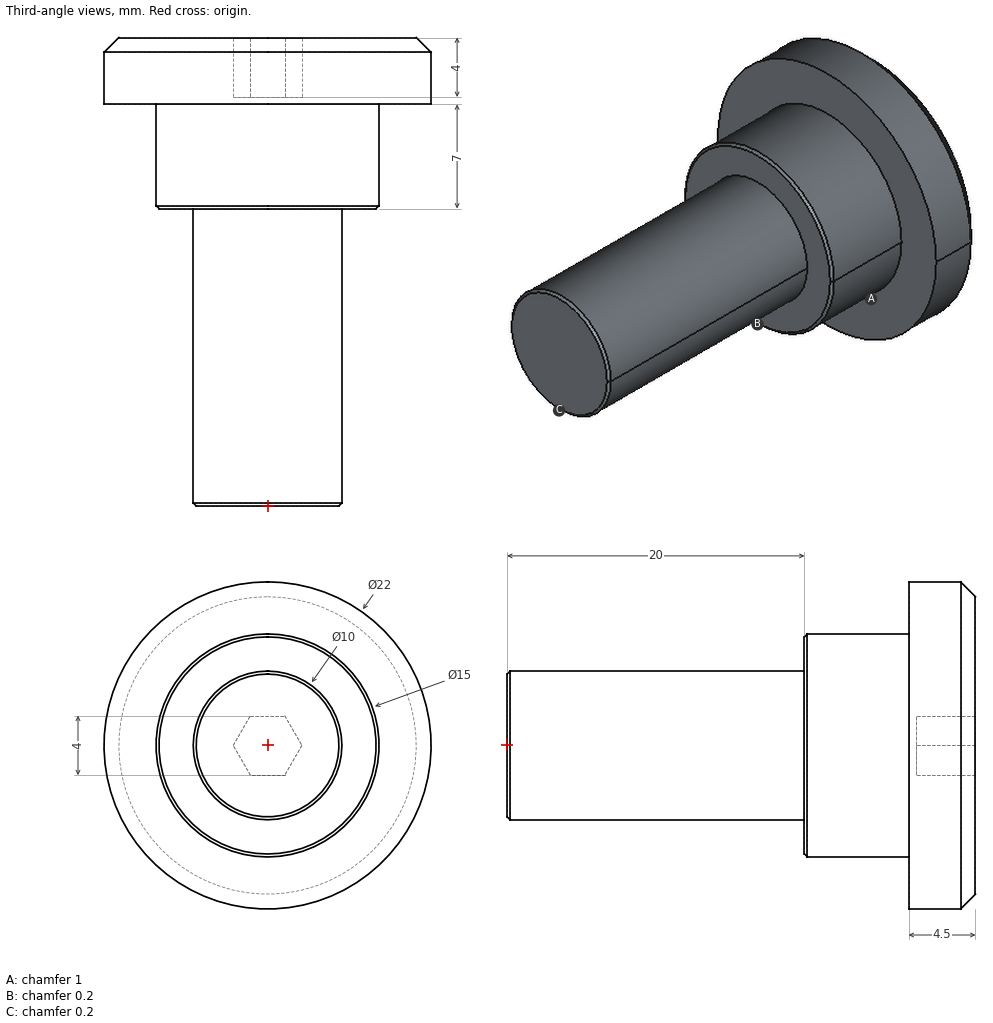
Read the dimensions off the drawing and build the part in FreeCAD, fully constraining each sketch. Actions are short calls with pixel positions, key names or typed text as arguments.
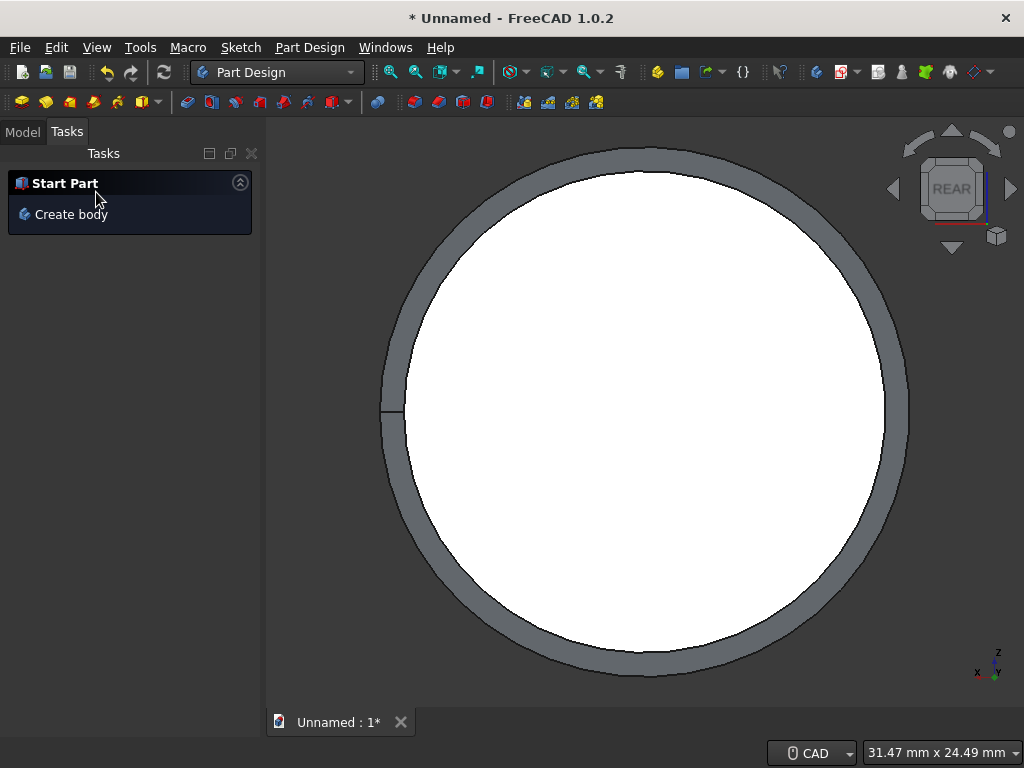
key(0)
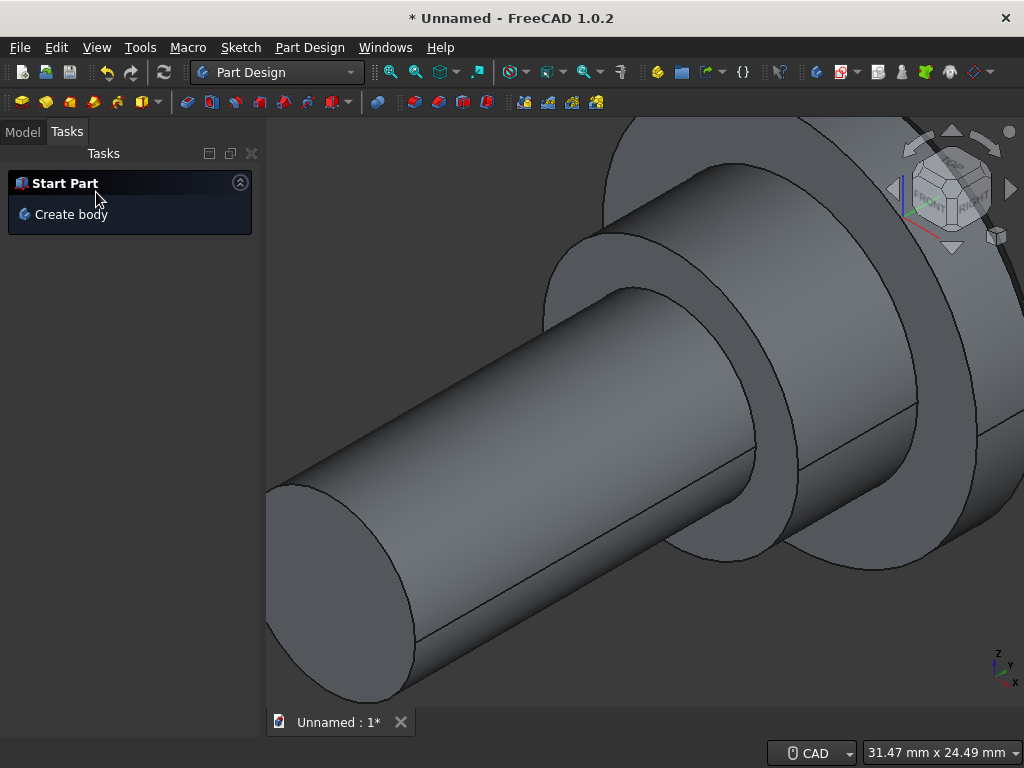
key(v)
key(f)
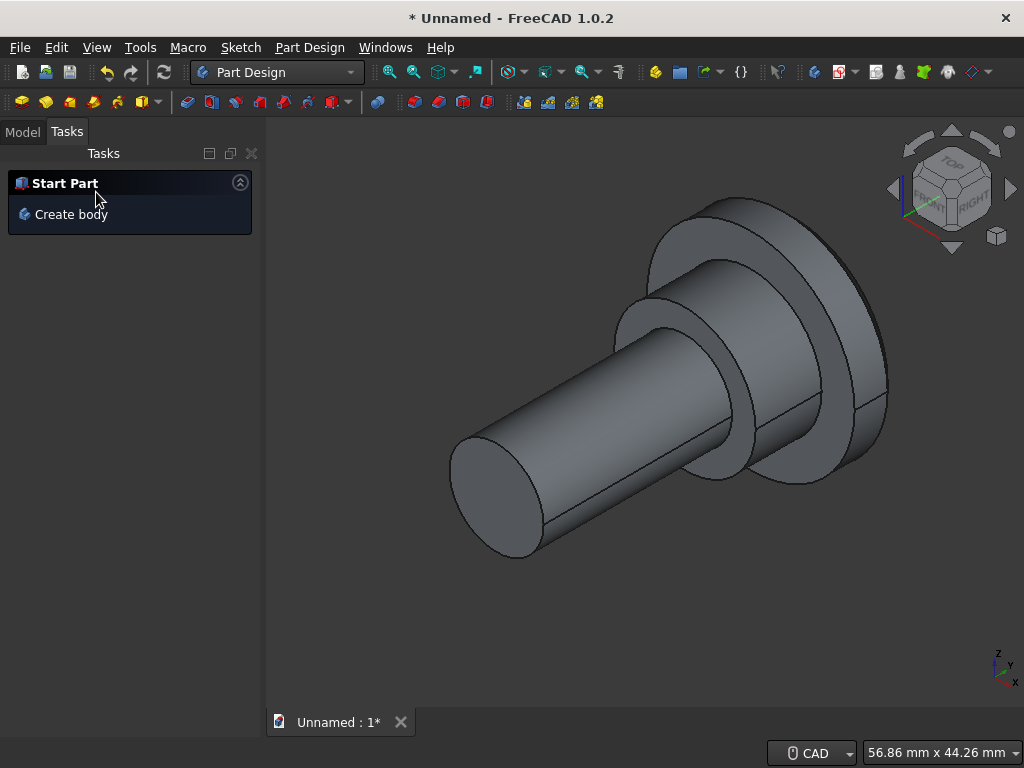
click(628, 307)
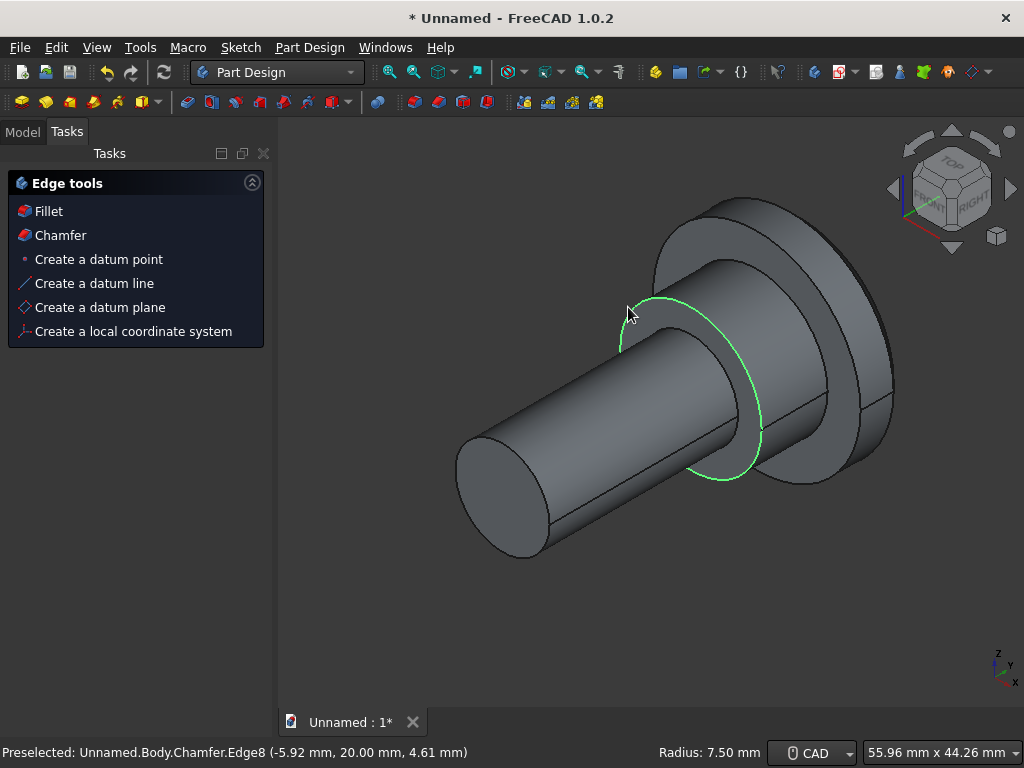
click(440, 102)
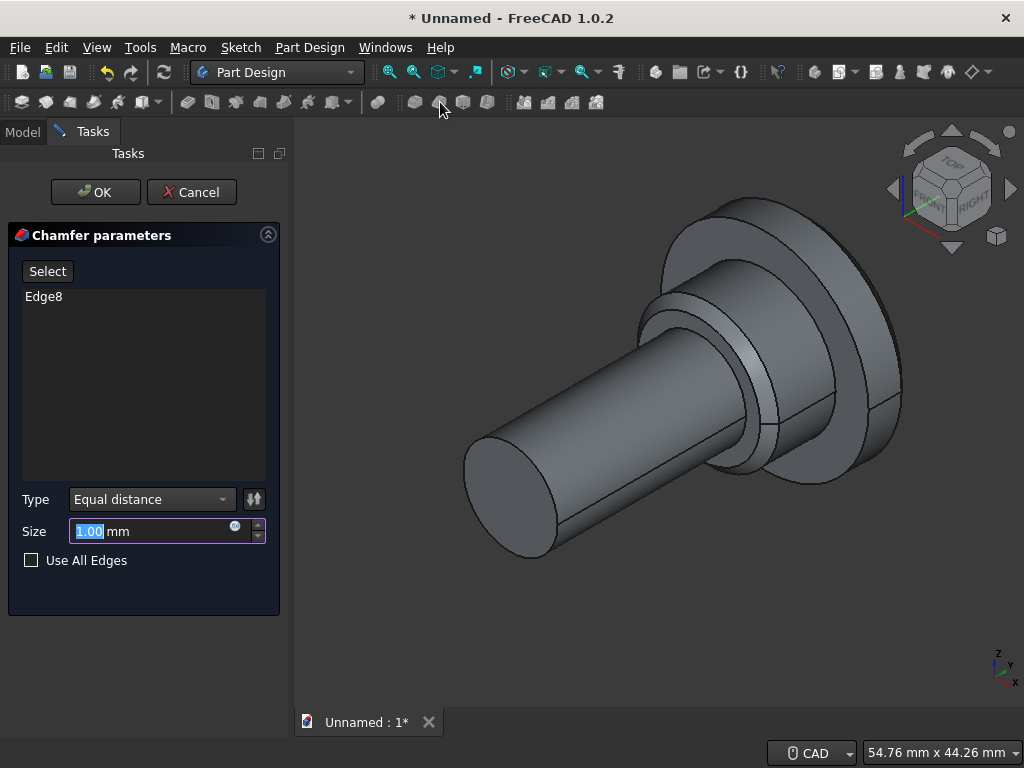
text(0.2)
key(Tab)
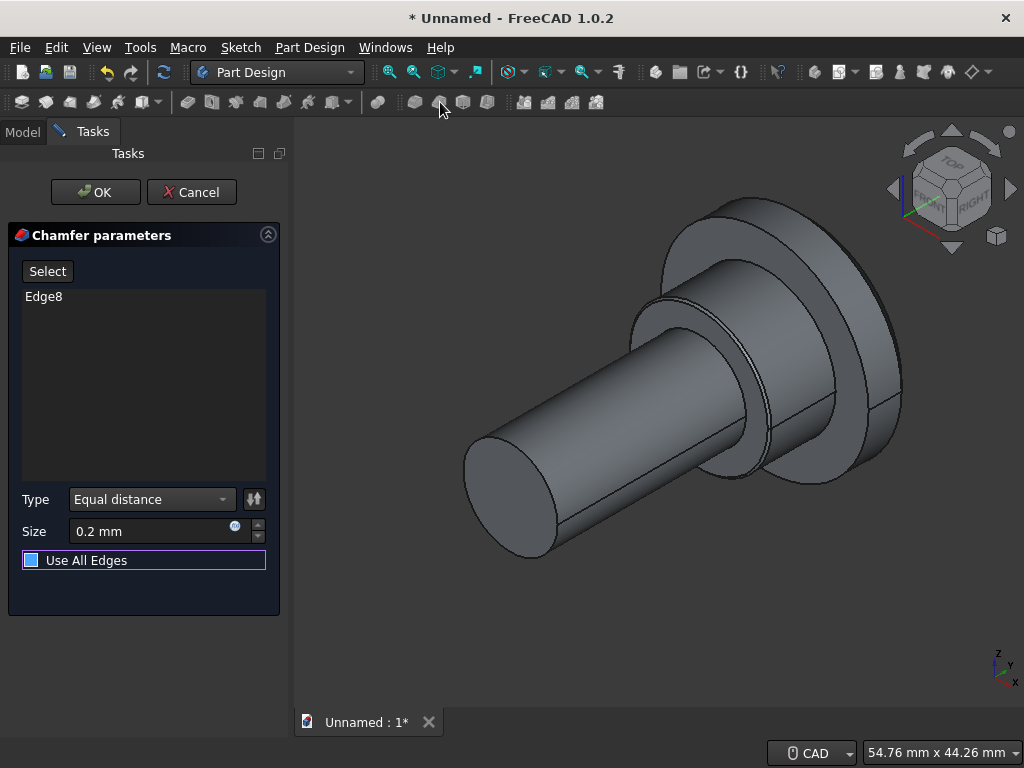
click(96, 192)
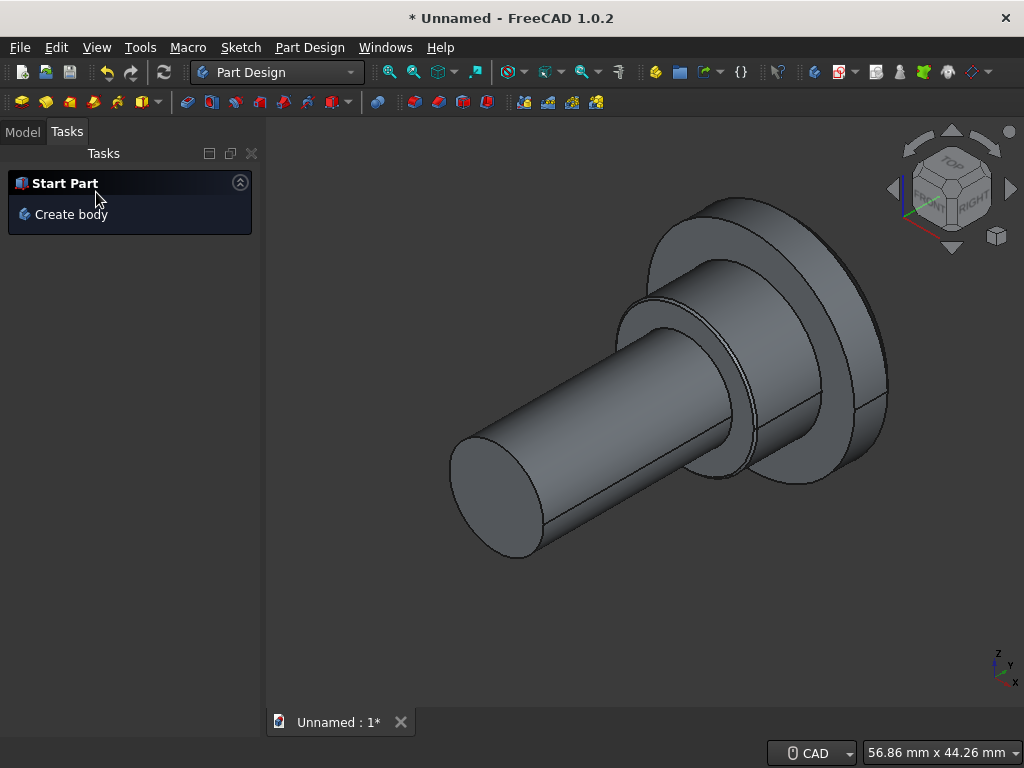
click(482, 436)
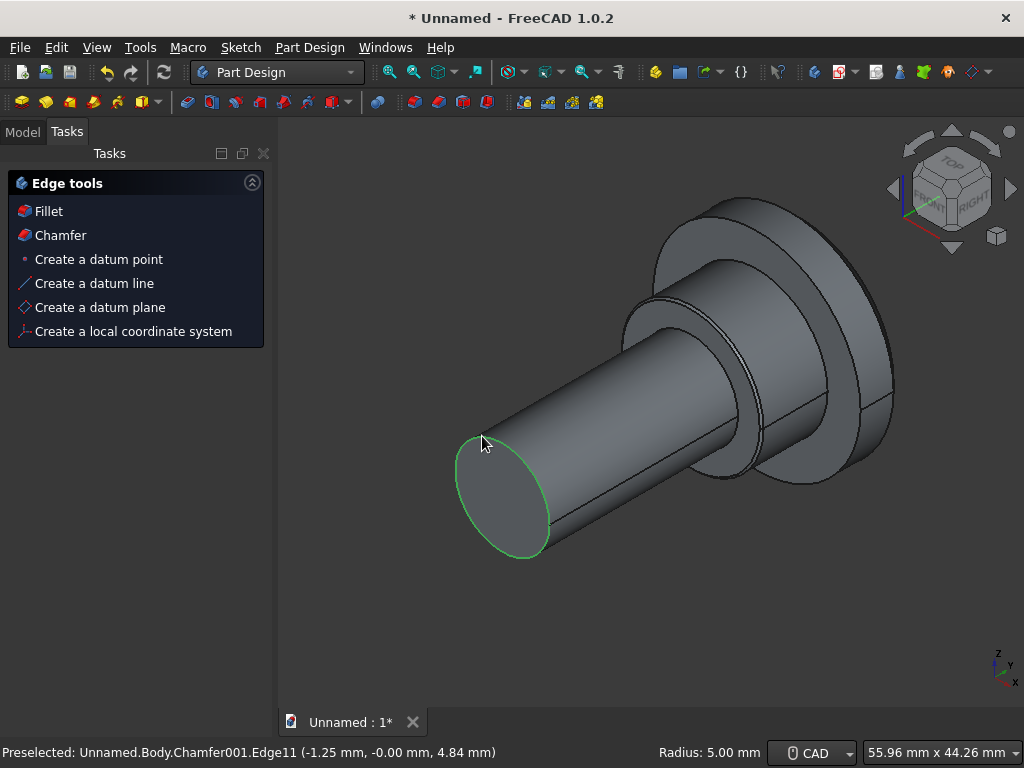
click(440, 102)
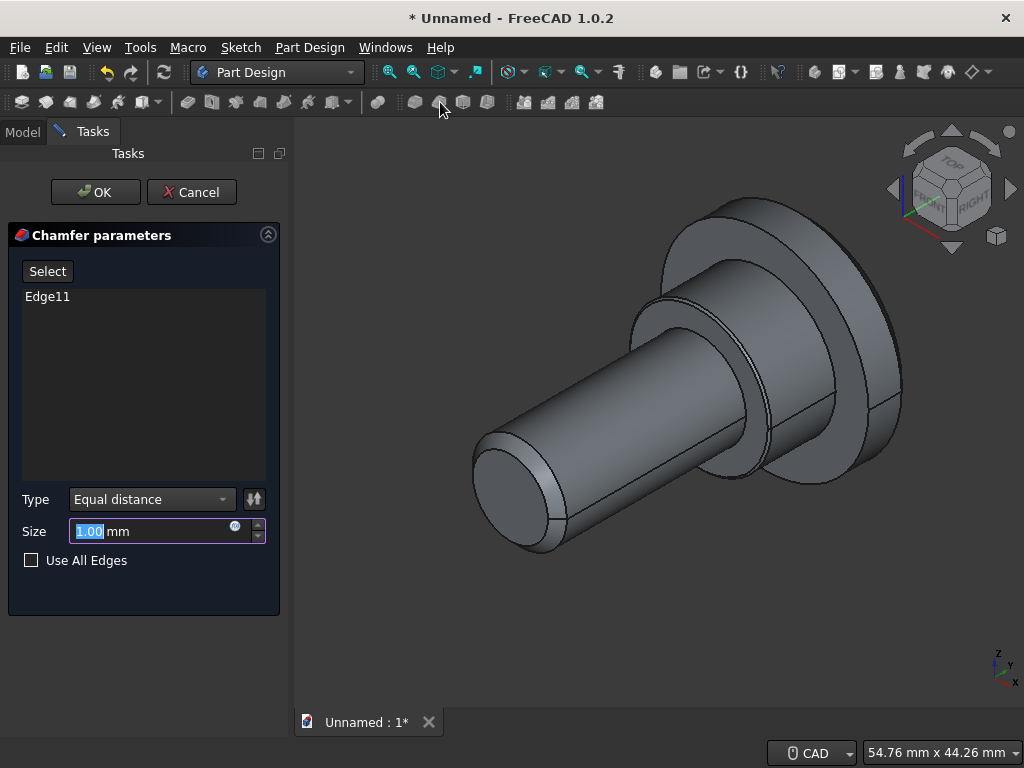
text(0.2)
key(Tab)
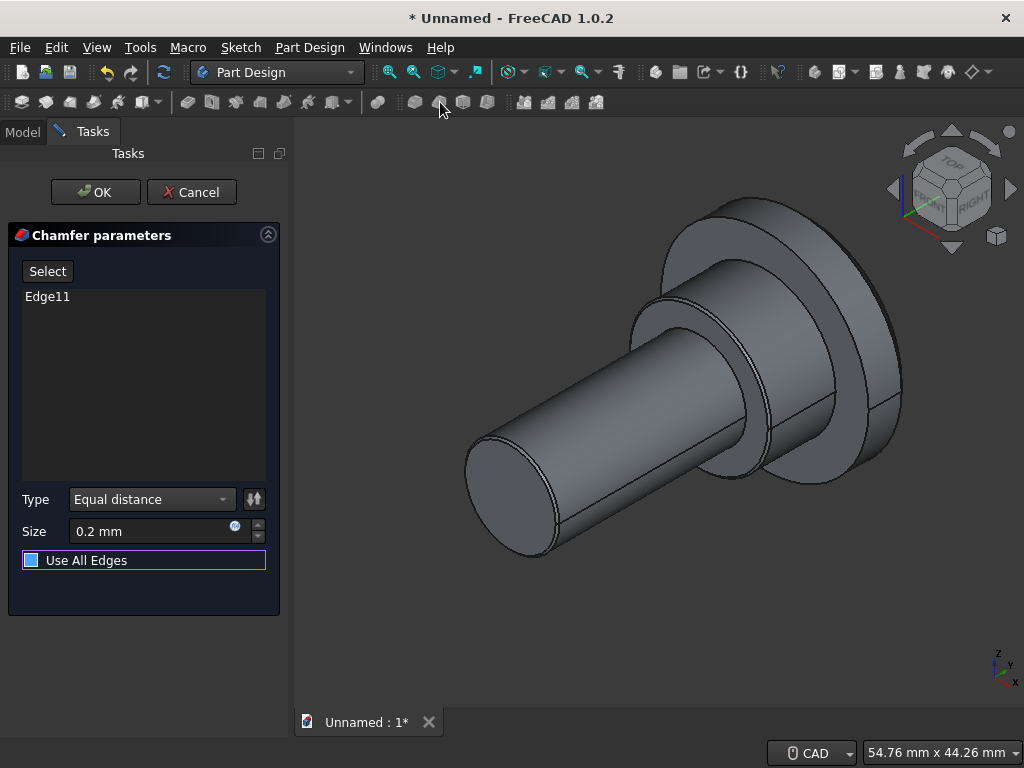
click(96, 192)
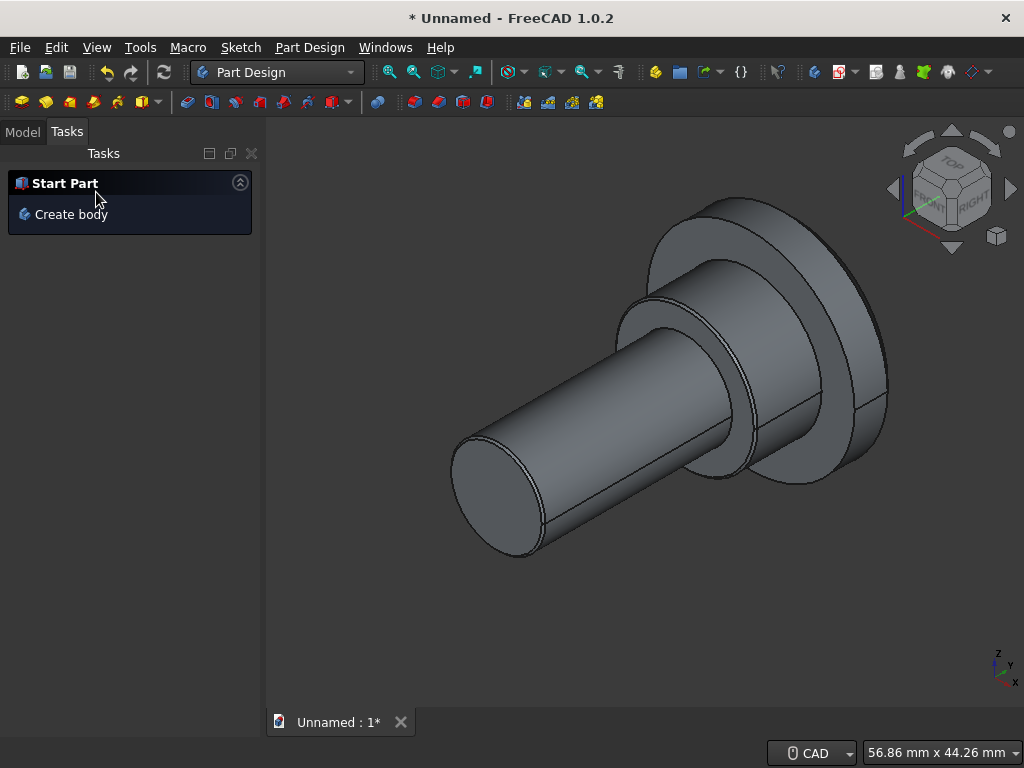
key(4)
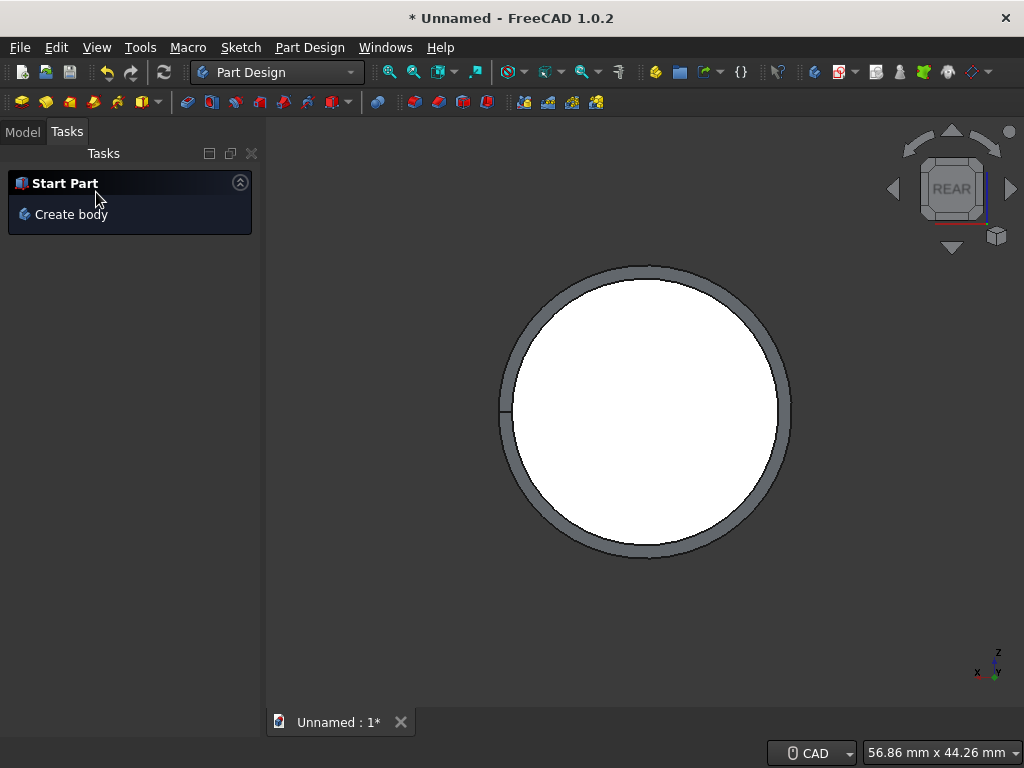
click(645, 411)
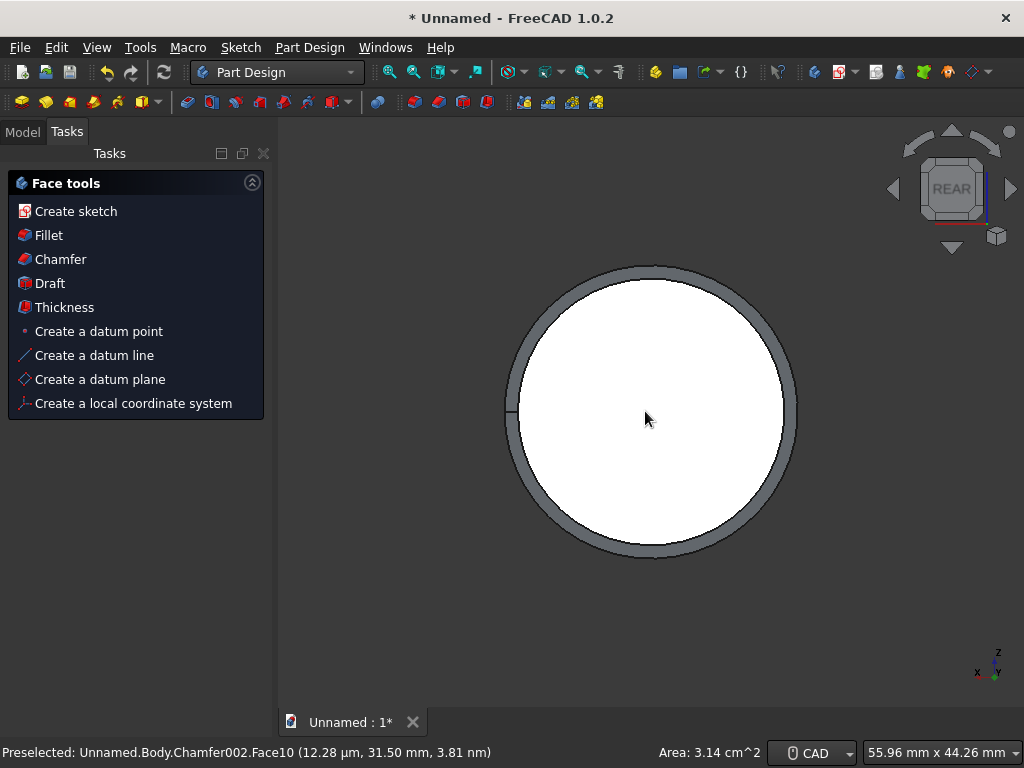
click(840, 72)